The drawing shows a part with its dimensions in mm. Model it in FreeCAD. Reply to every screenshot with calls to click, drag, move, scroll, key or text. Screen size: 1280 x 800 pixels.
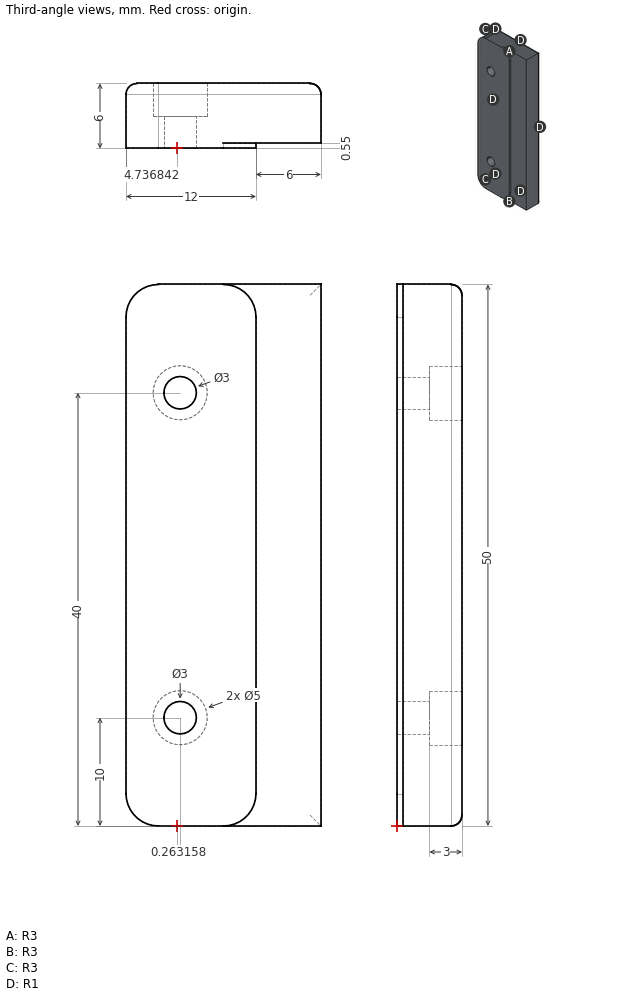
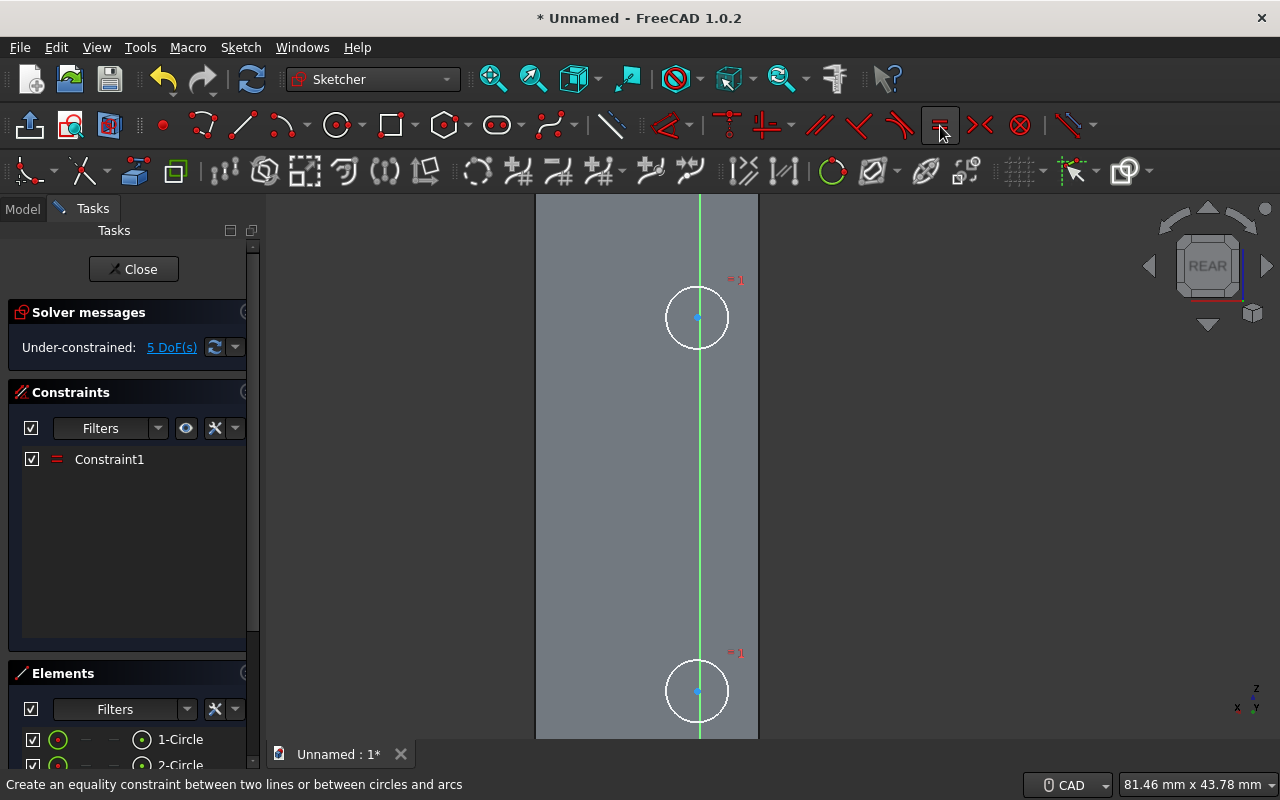
click(719, 669)
click(741, 646)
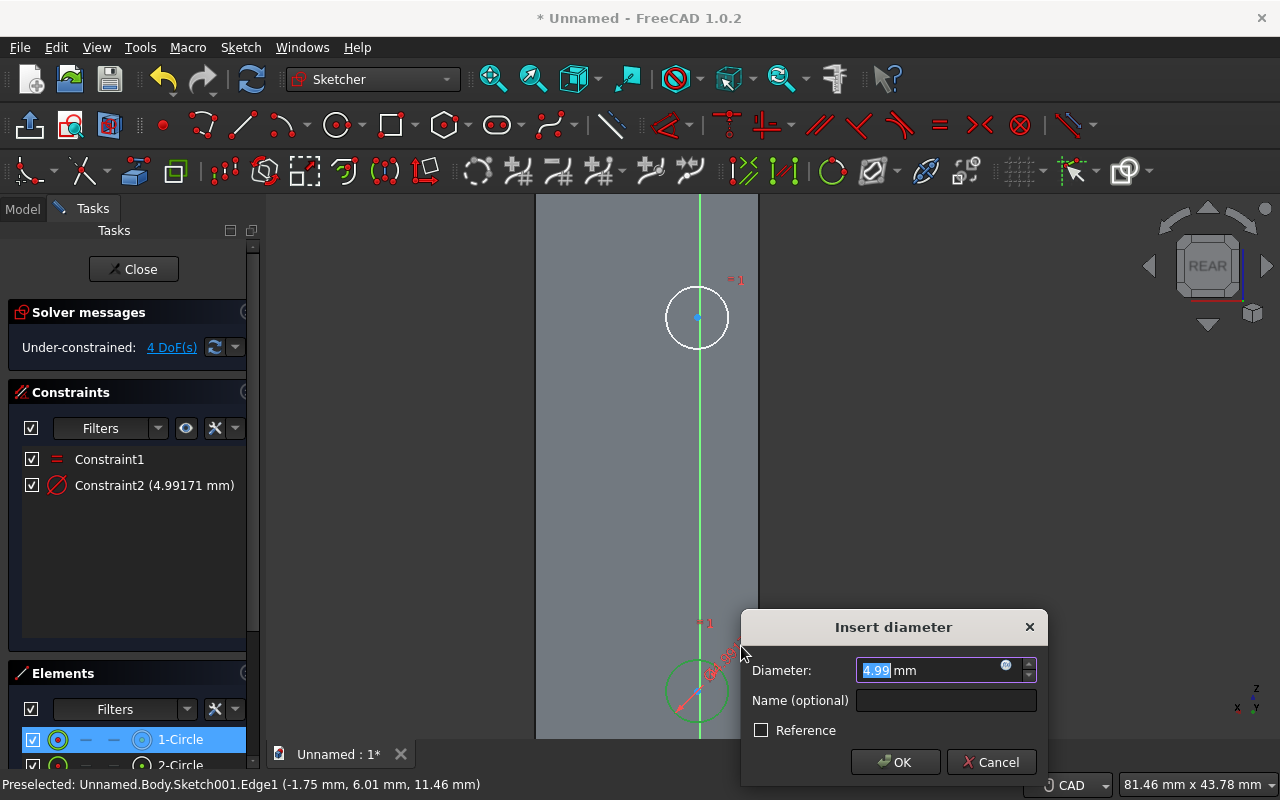
text(5)
key(Return)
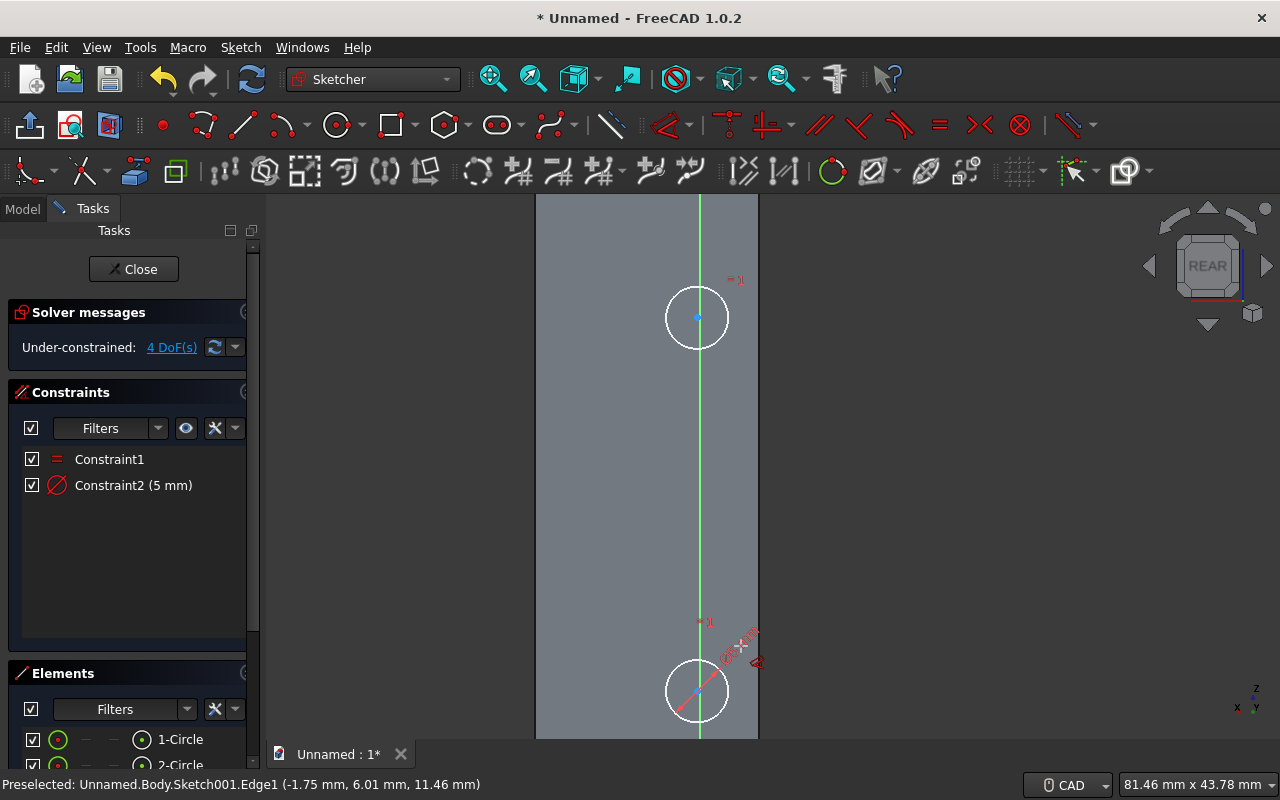
click(697, 691)
click(758, 701)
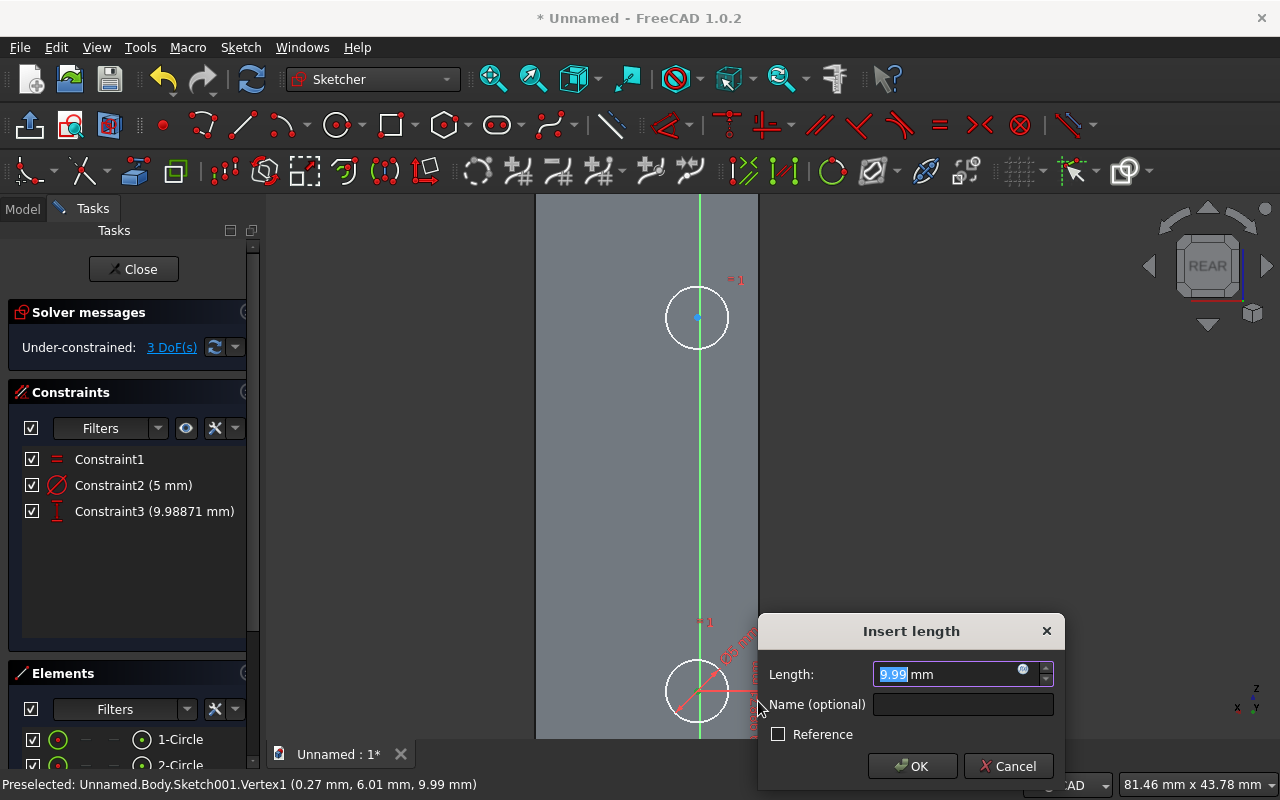
text(10)
key(Return)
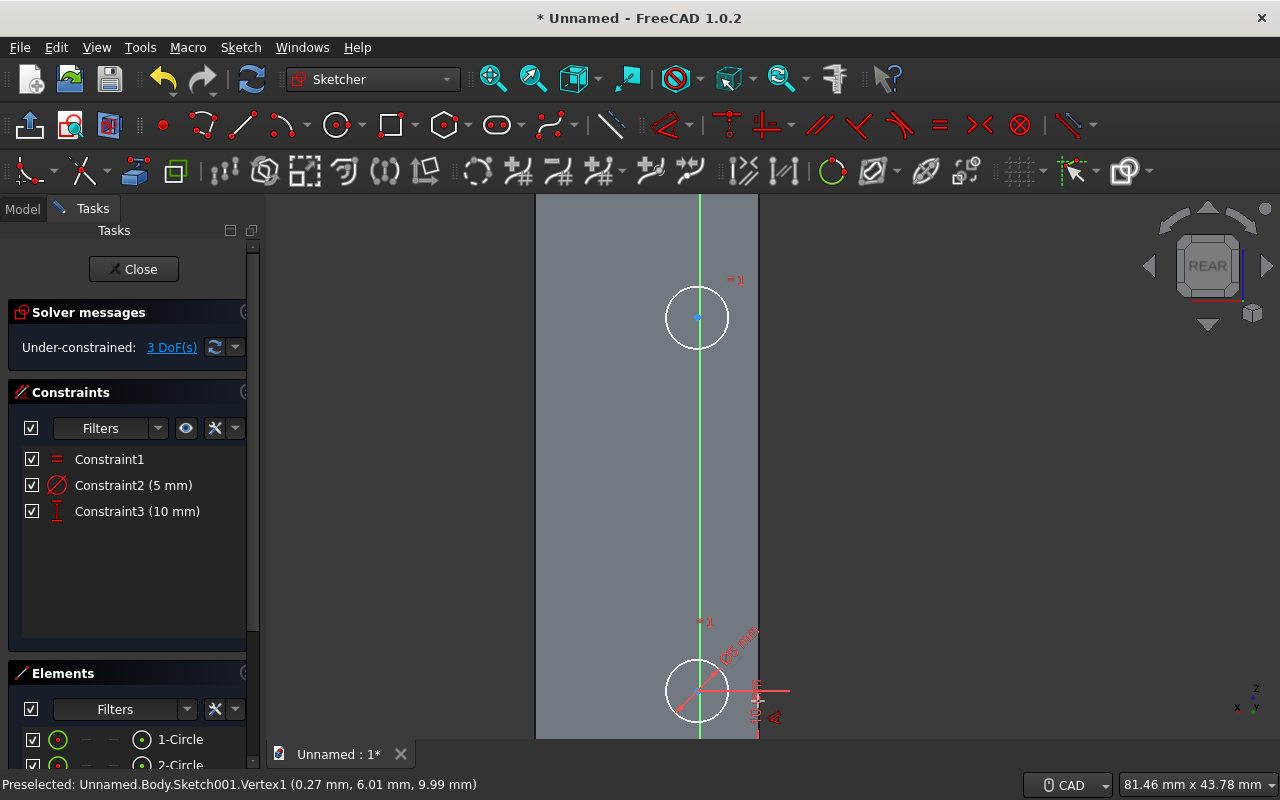
click(697, 318)
click(734, 514)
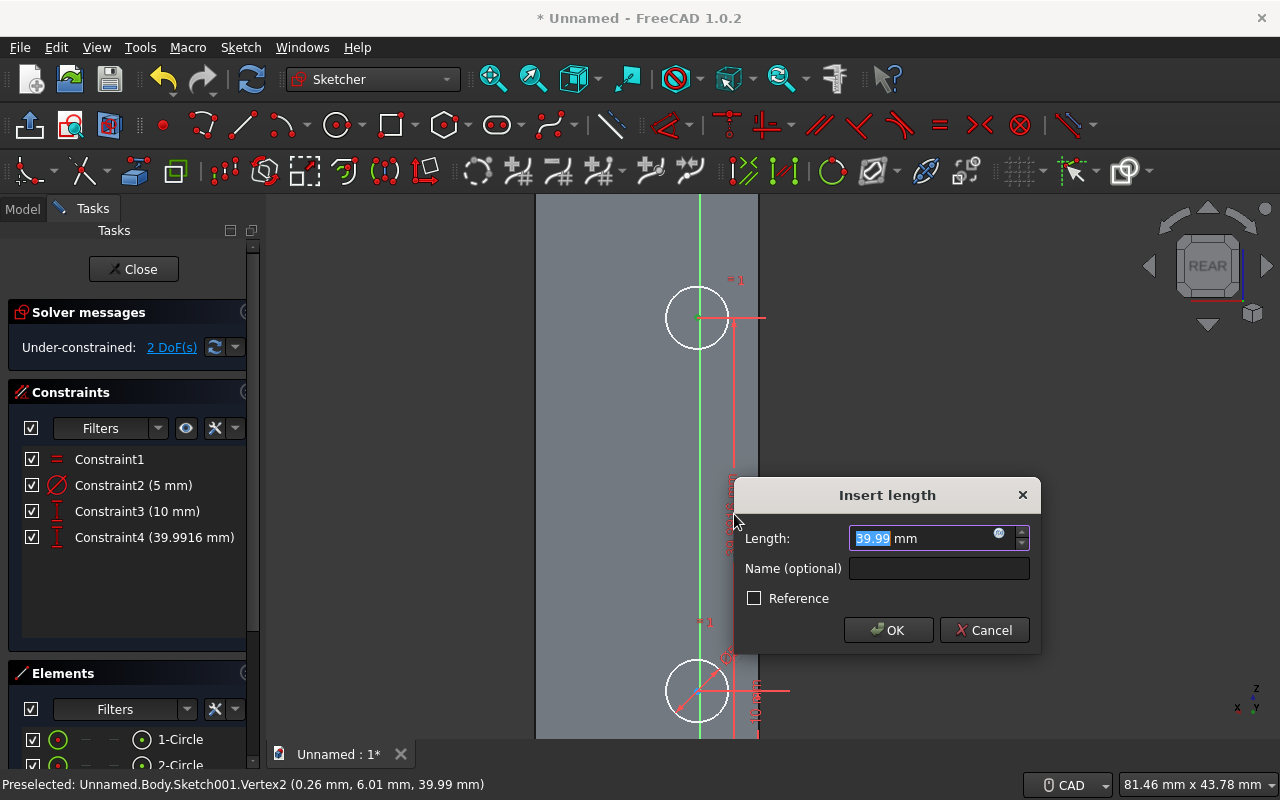
text(40)
key(Return)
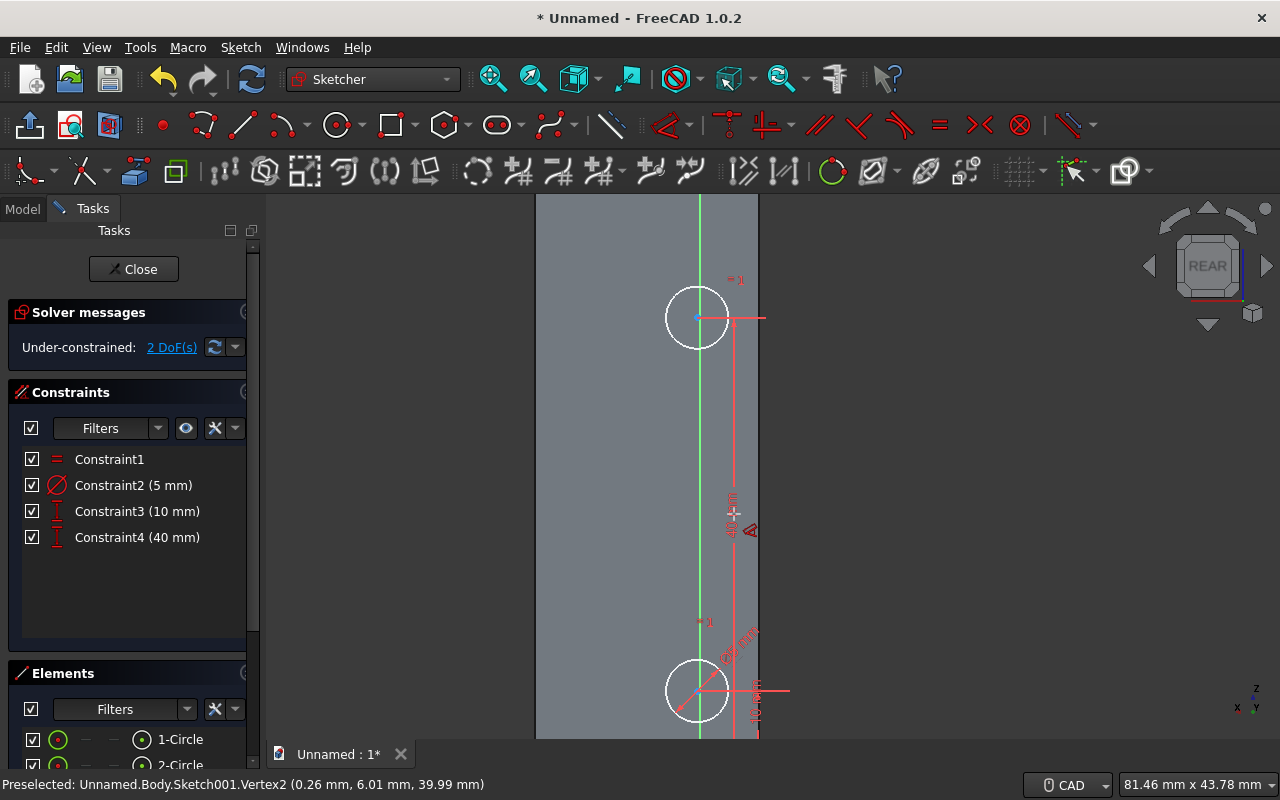
scroll(697, 691, up, 13)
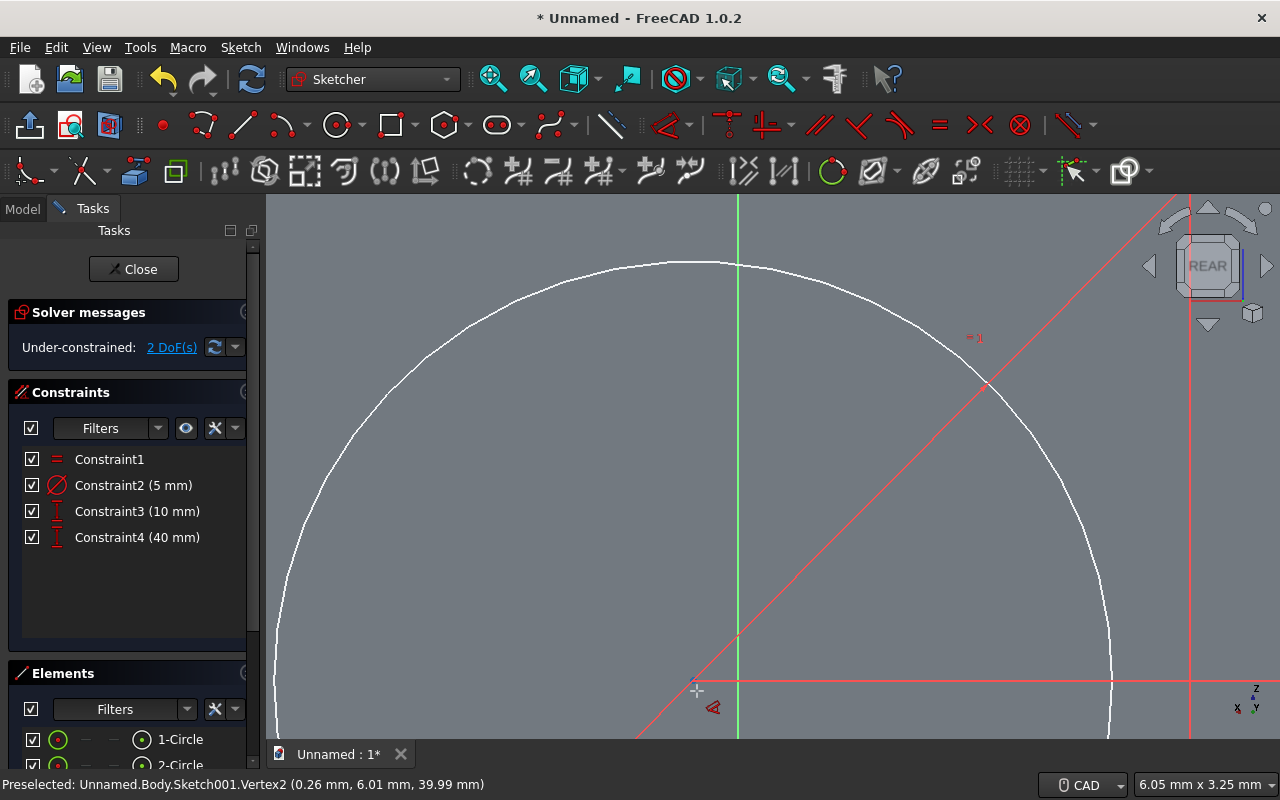
click(693, 681)
click(715, 647)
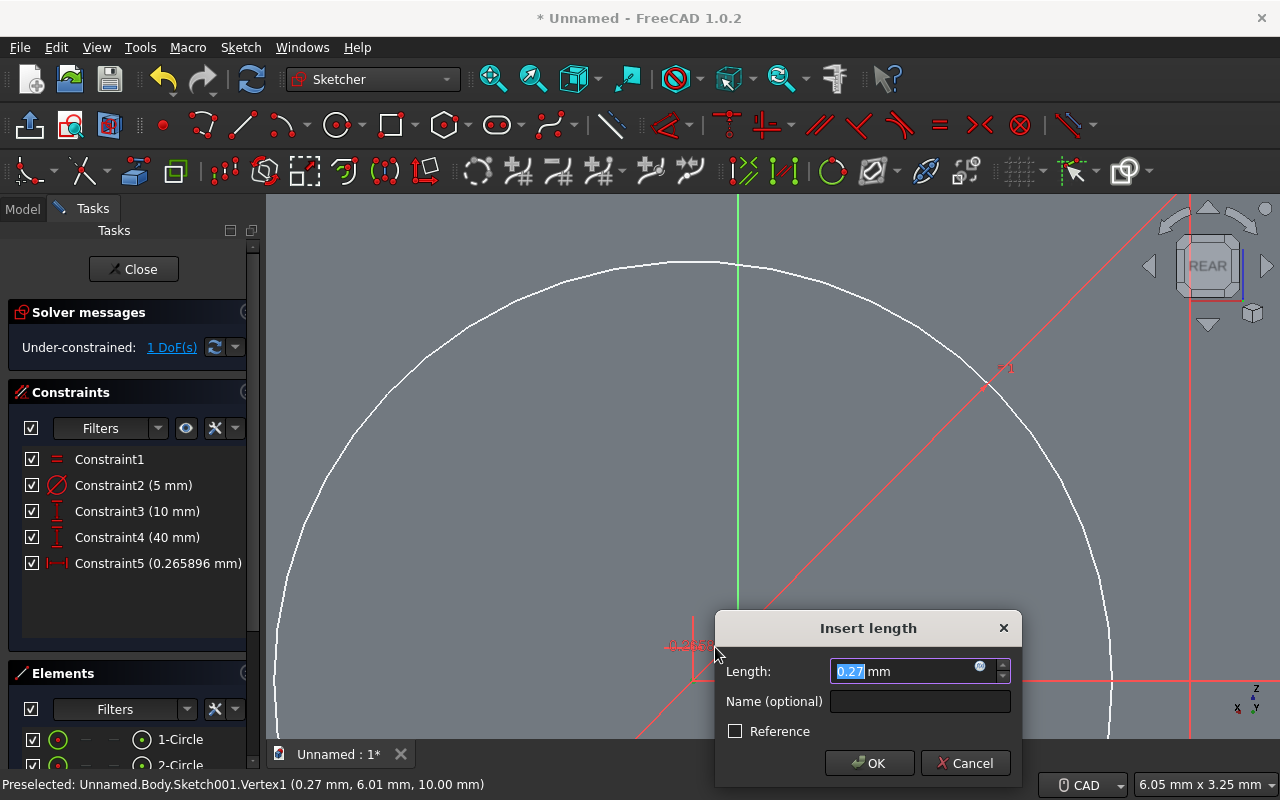
text(0.263158)
key(Return)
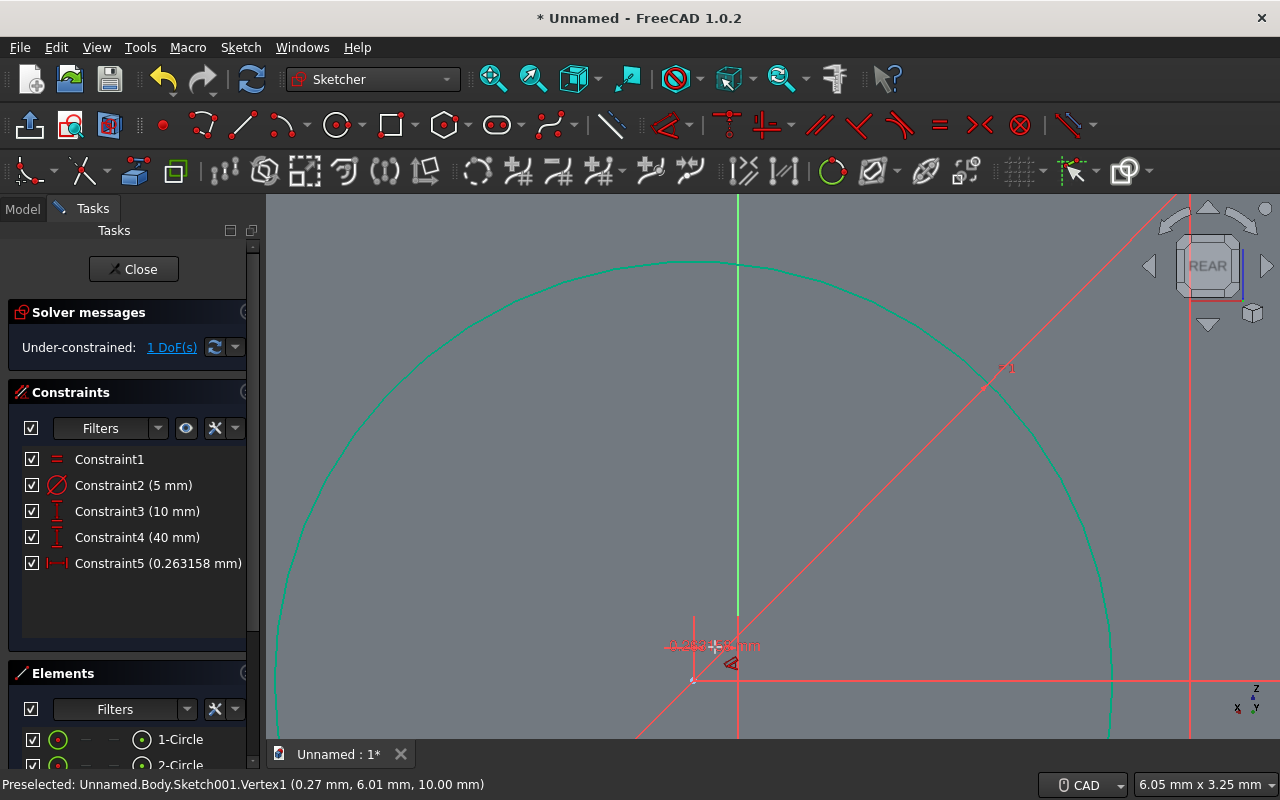
scroll(705, 554, down, 15)